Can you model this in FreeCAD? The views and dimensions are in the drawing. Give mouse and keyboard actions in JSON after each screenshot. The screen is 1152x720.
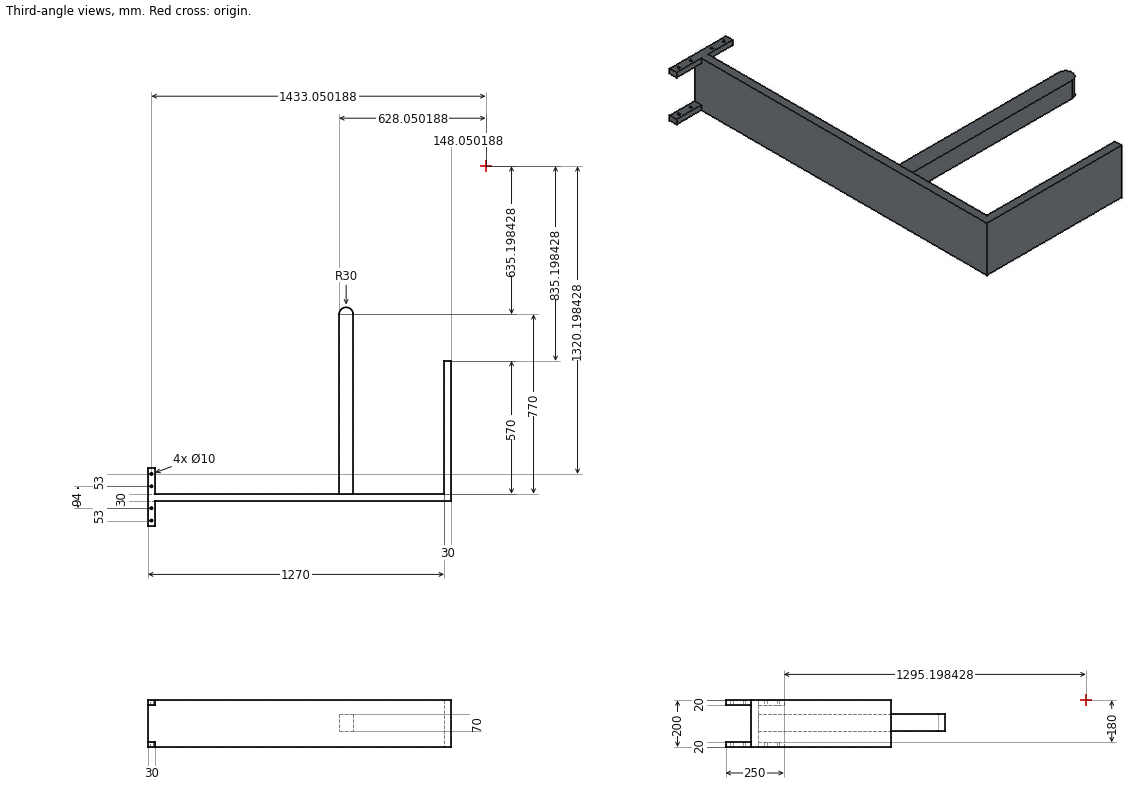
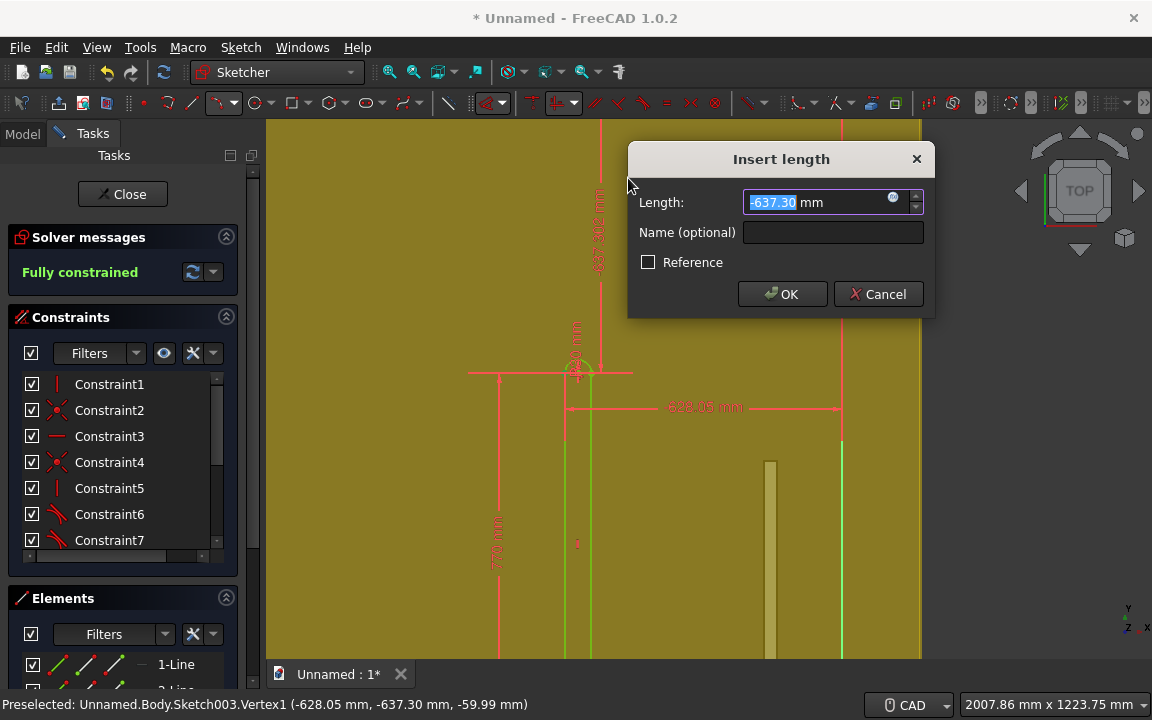
{"action": "type", "text": "-635.198428"}
{"action": "key", "text": "Return"}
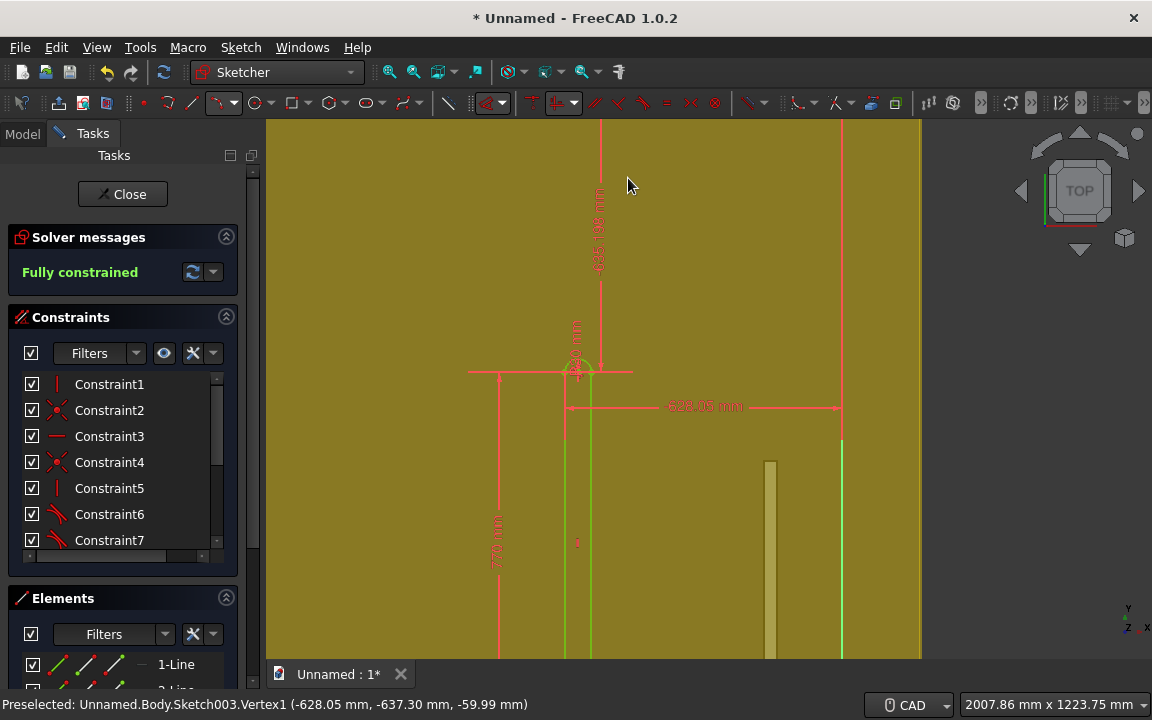
{"action": "left_click", "coordinate": [123, 194]}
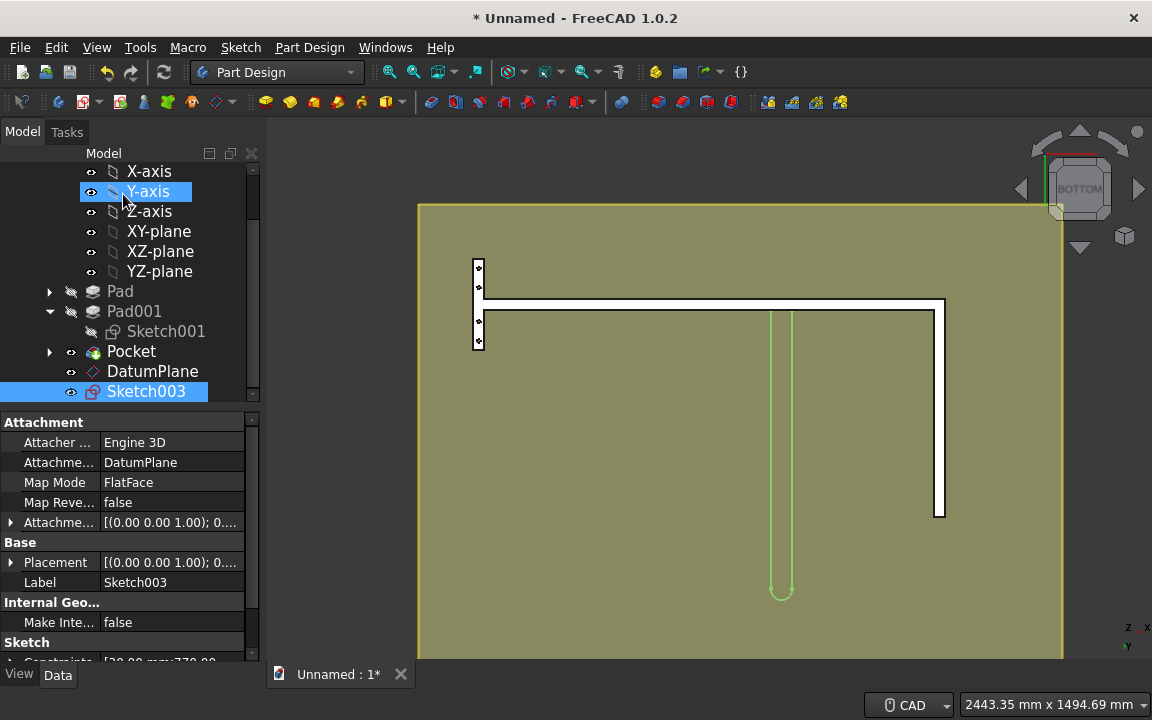
{"action": "left_click", "coordinate": [266, 102]}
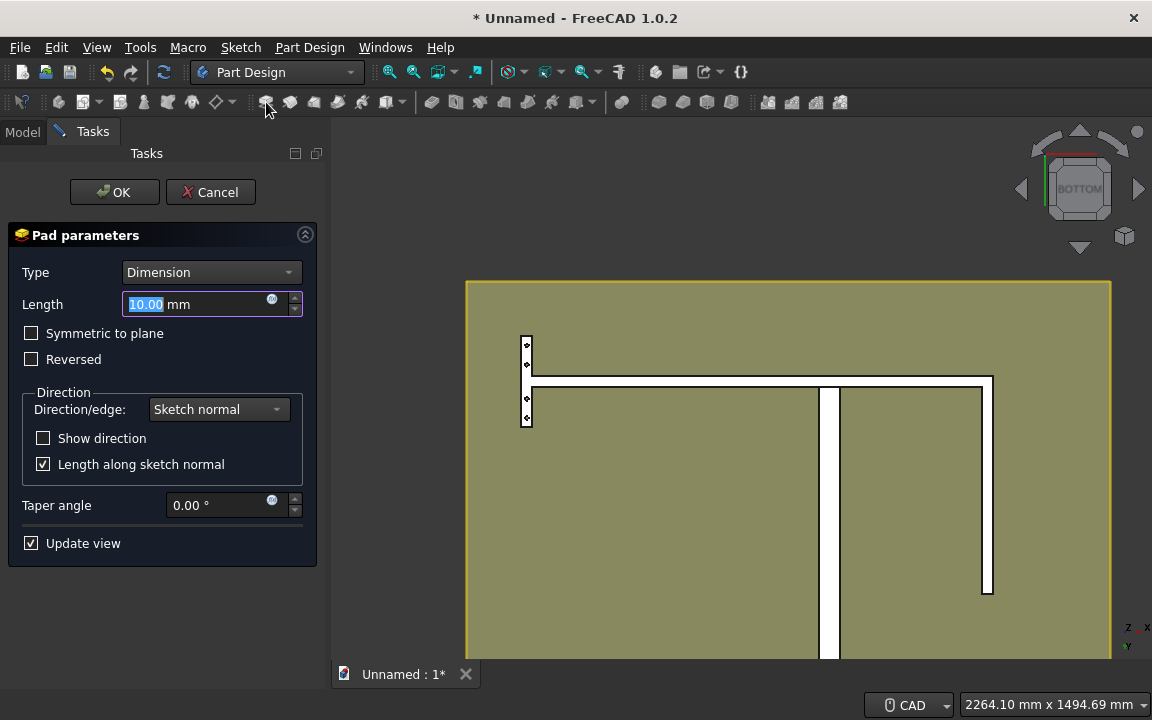
{"action": "type", "text": "70"}
{"action": "key", "text": "Tab"}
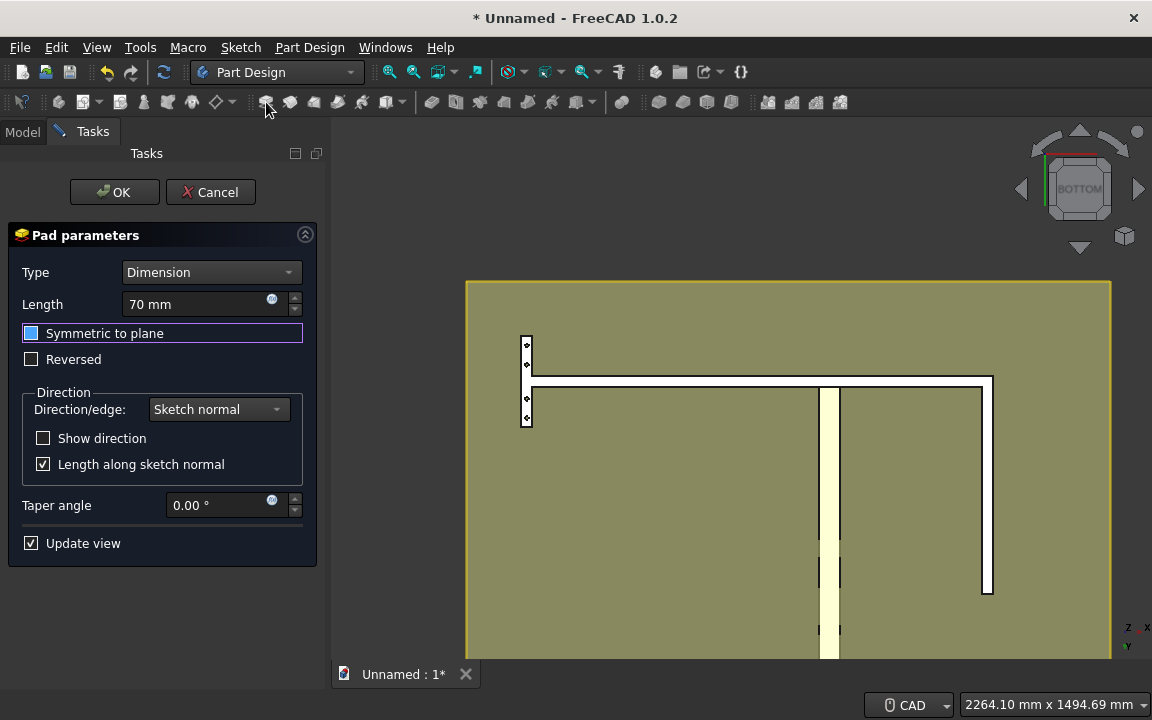
{"action": "left_click", "coordinate": [30, 359]}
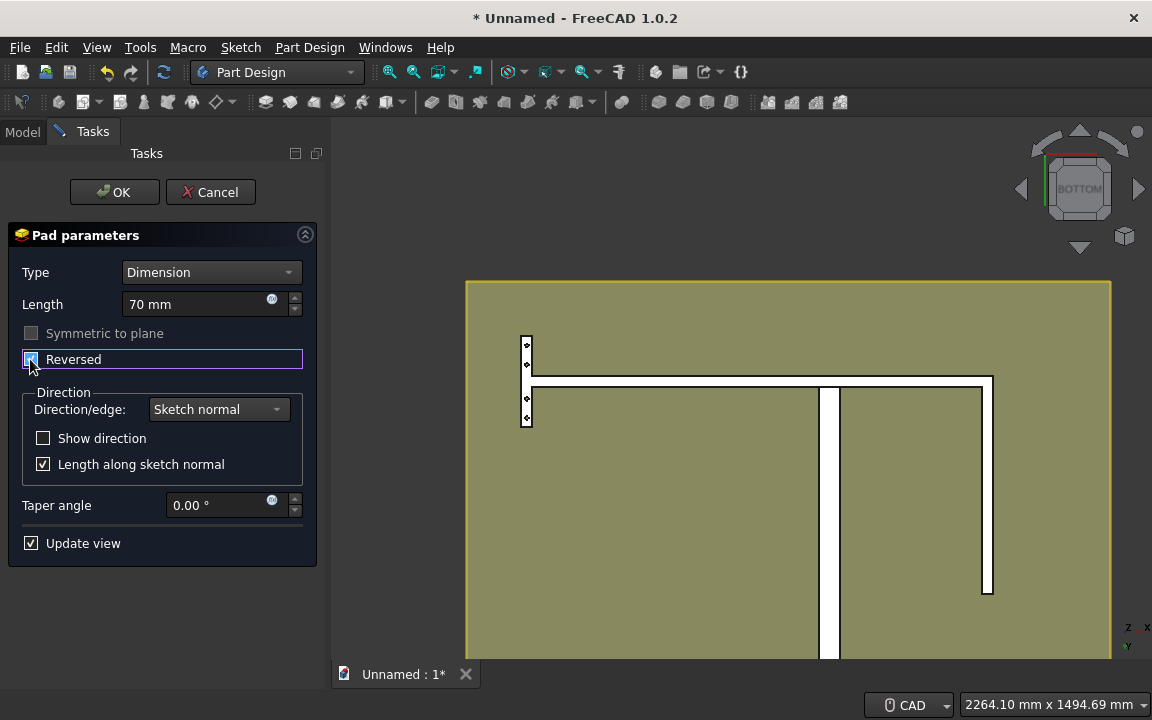
{"action": "left_click", "coordinate": [115, 192]}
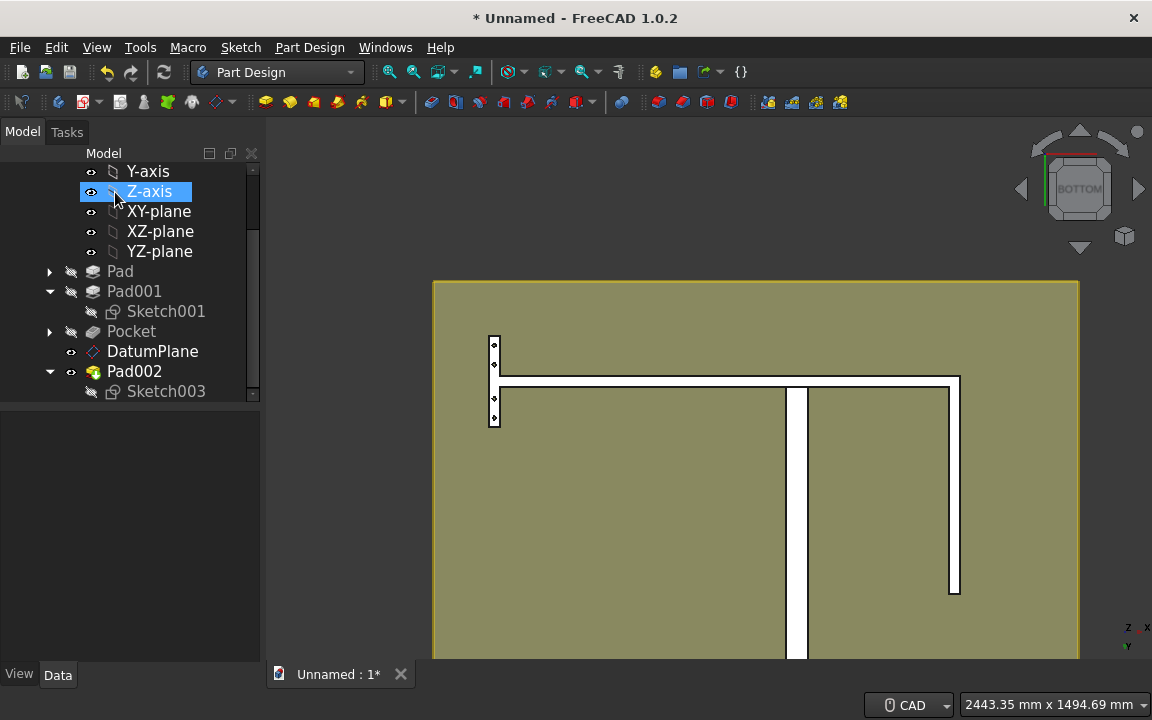
{"action": "left_click", "coordinate": [116, 352]}
{"action": "key", "text": "space"}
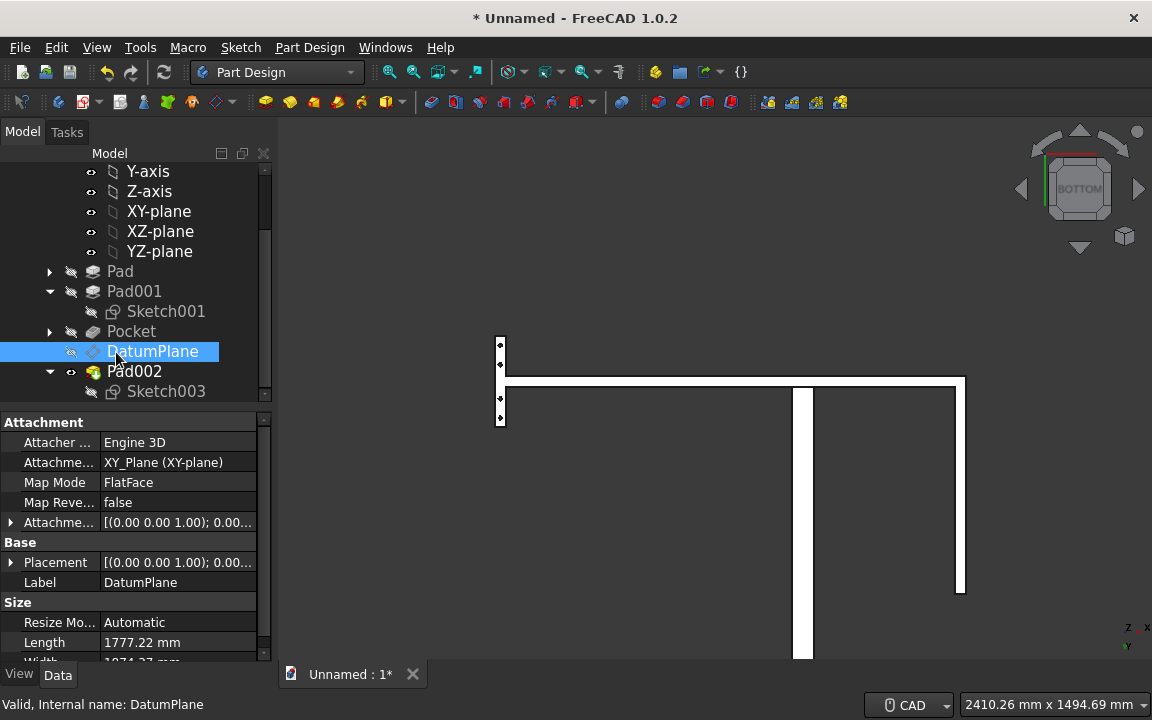
{"action": "key", "text": "0"}